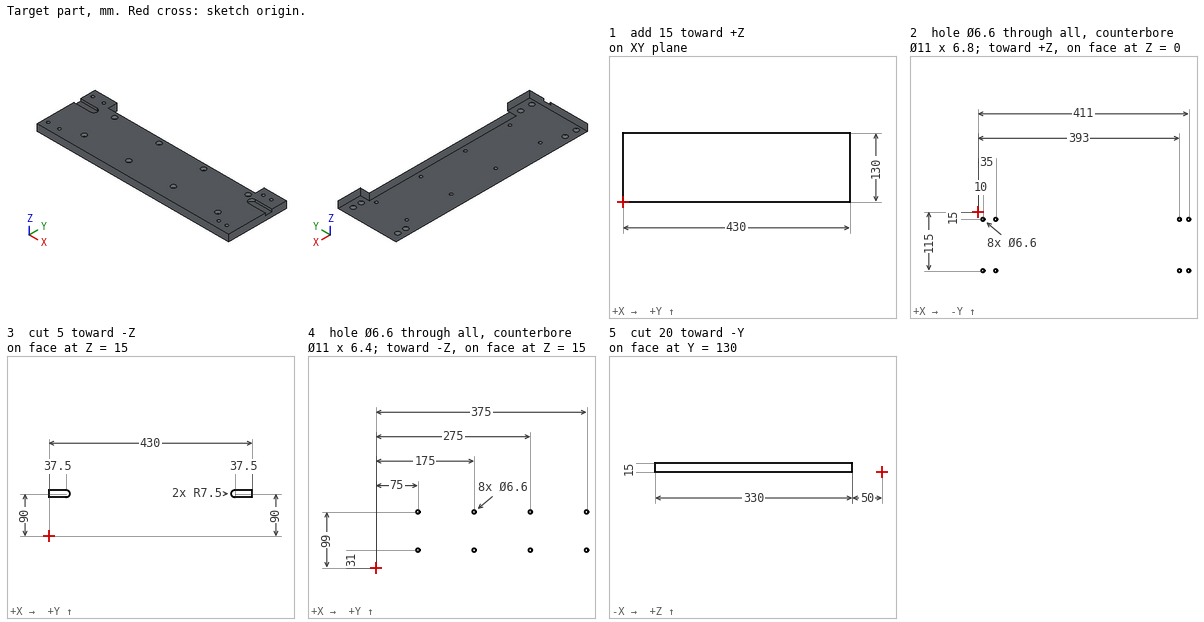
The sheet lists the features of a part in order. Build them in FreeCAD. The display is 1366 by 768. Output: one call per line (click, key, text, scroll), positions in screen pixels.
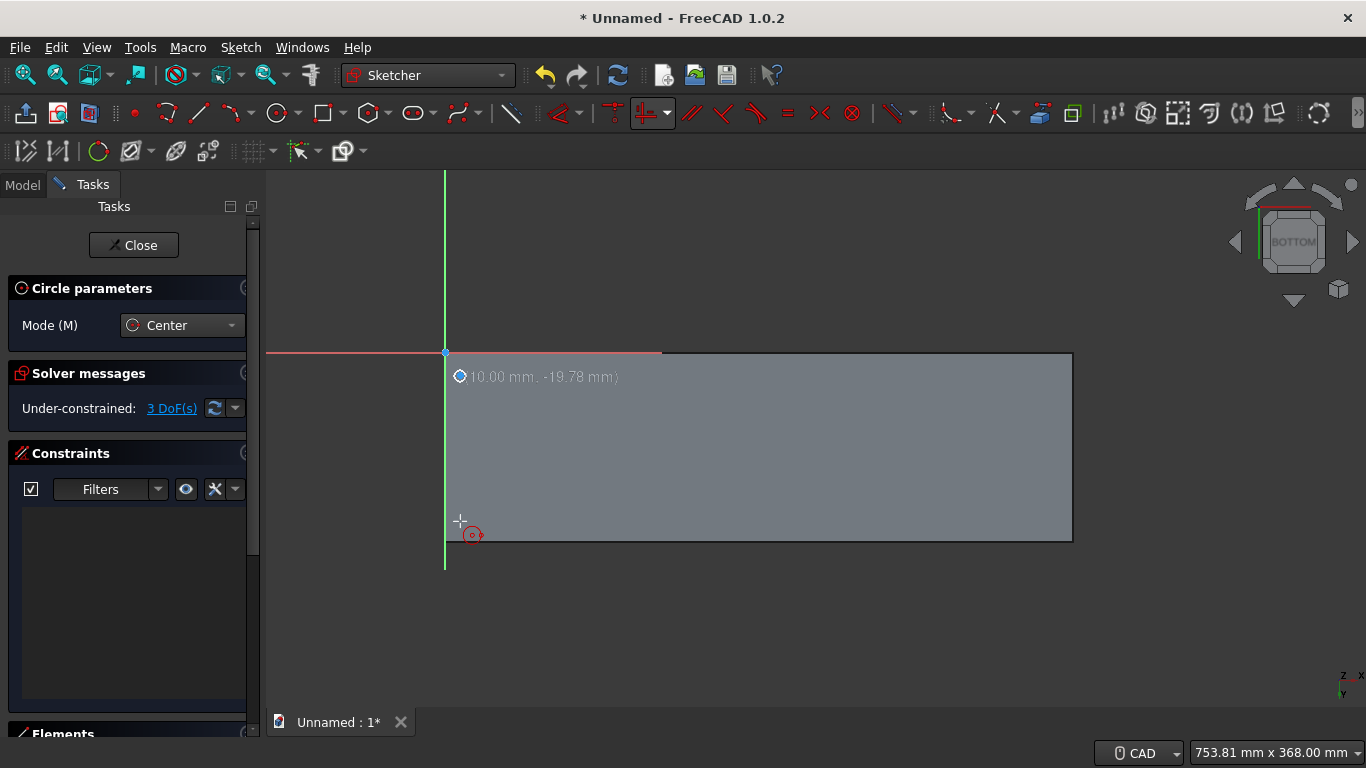
click(460, 521)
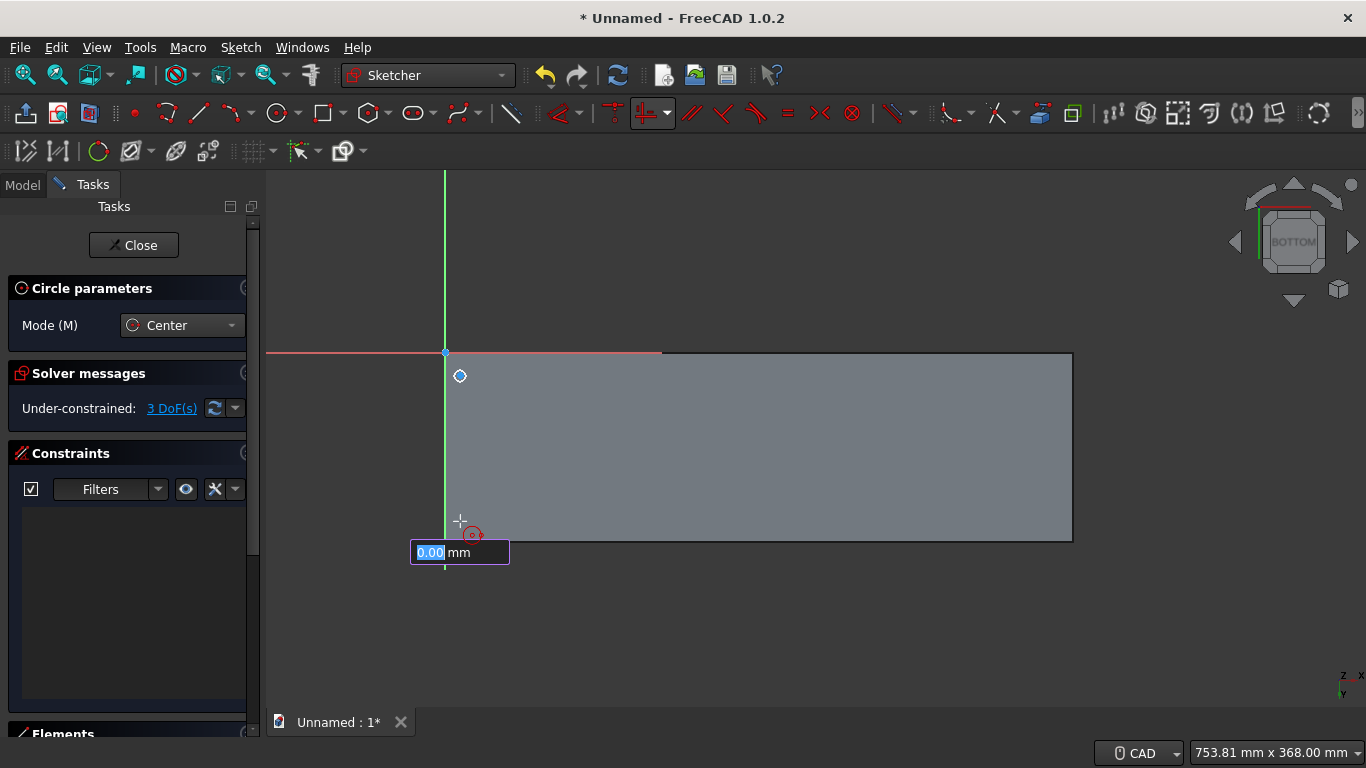
scroll(463, 517, up, 6)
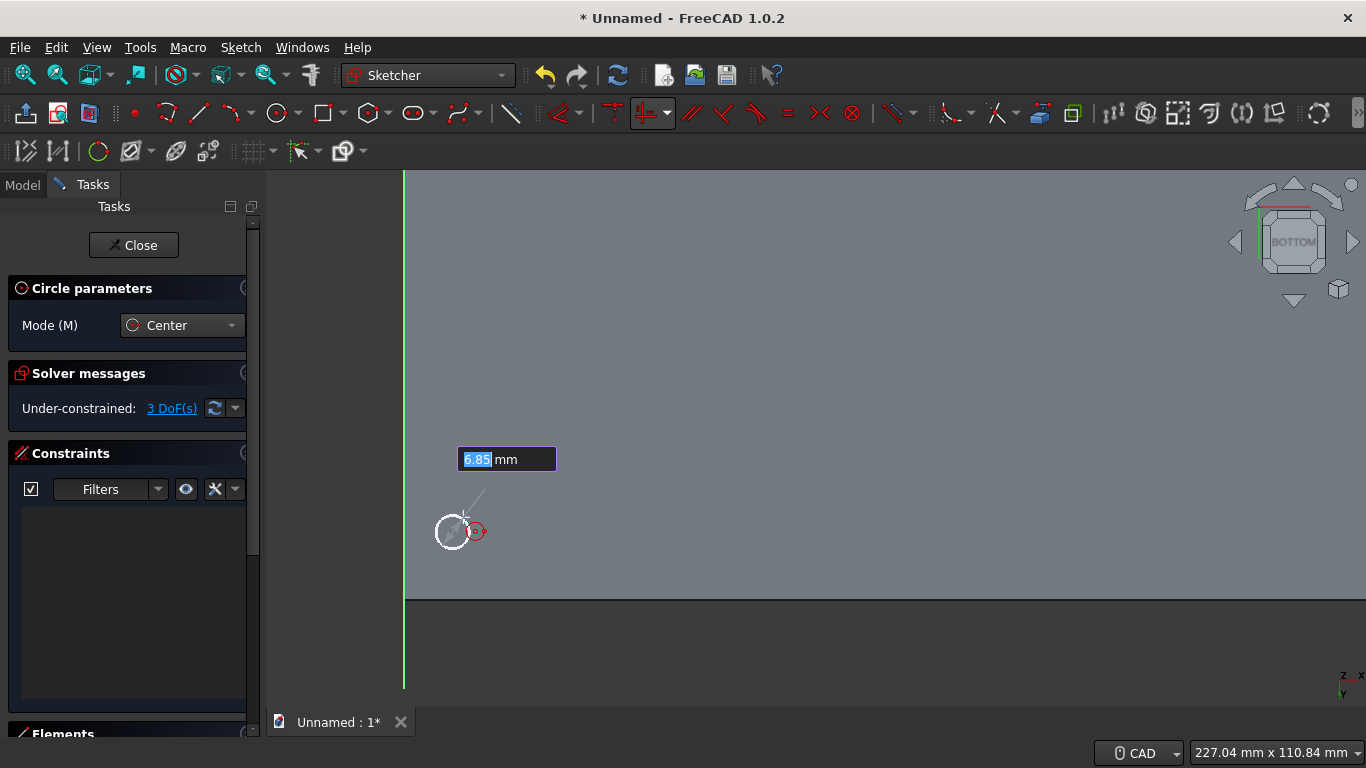
click(464, 516)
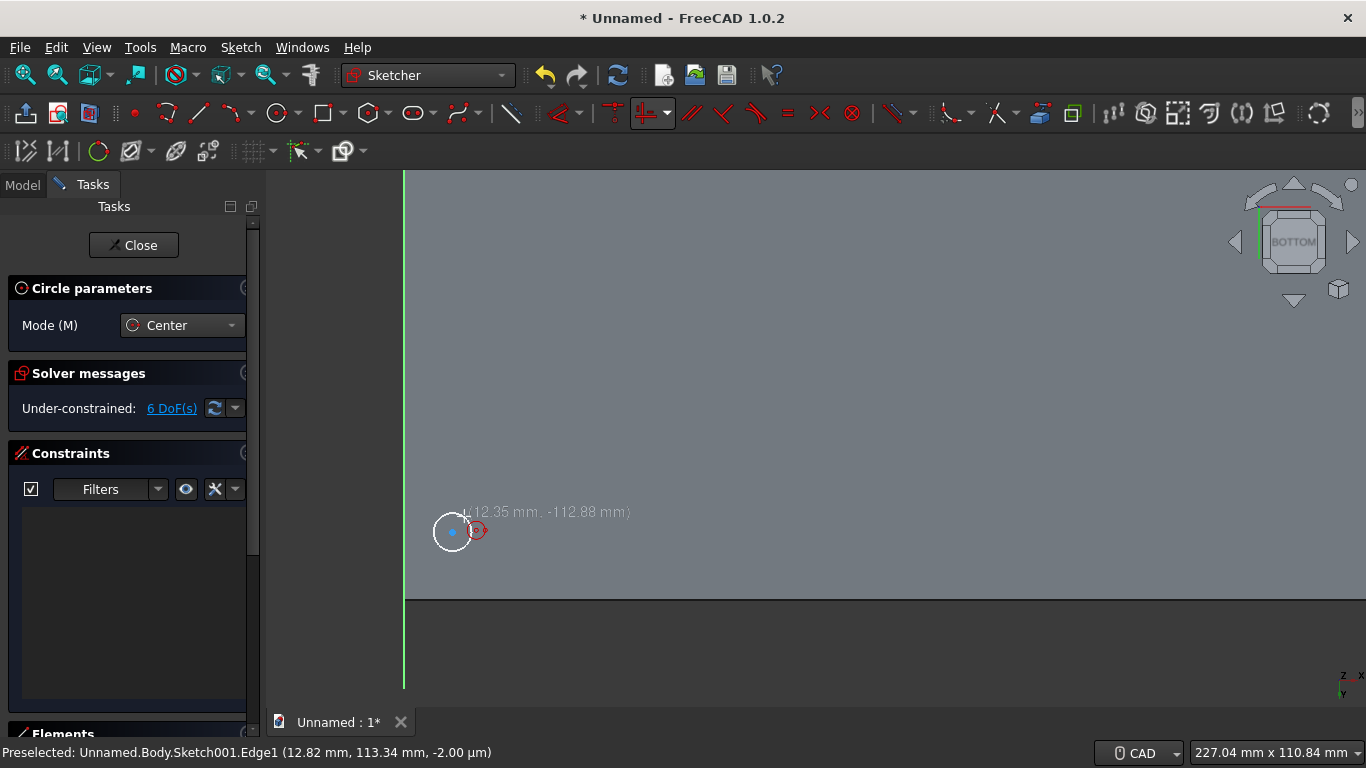
scroll(463, 517, down, 6)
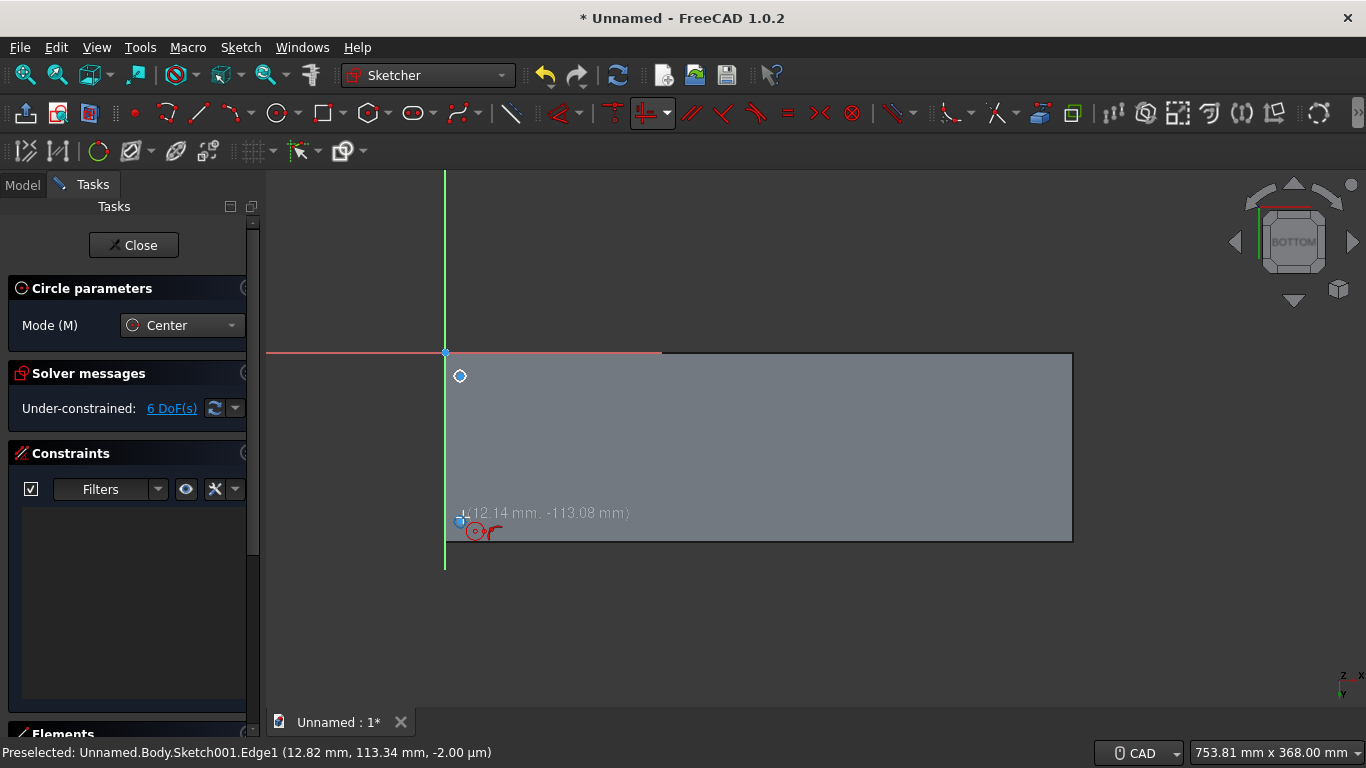
scroll(496, 375, up, 8)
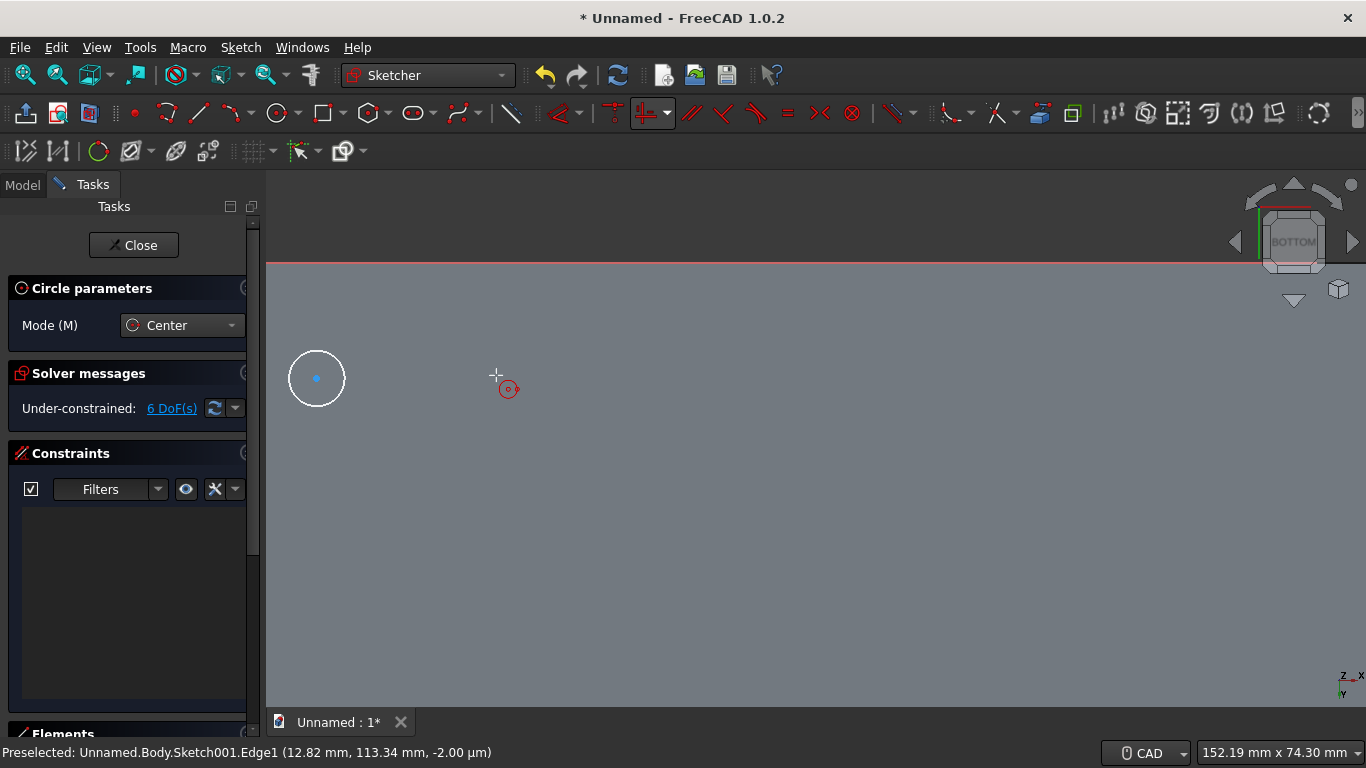
scroll(496, 375, down, 8)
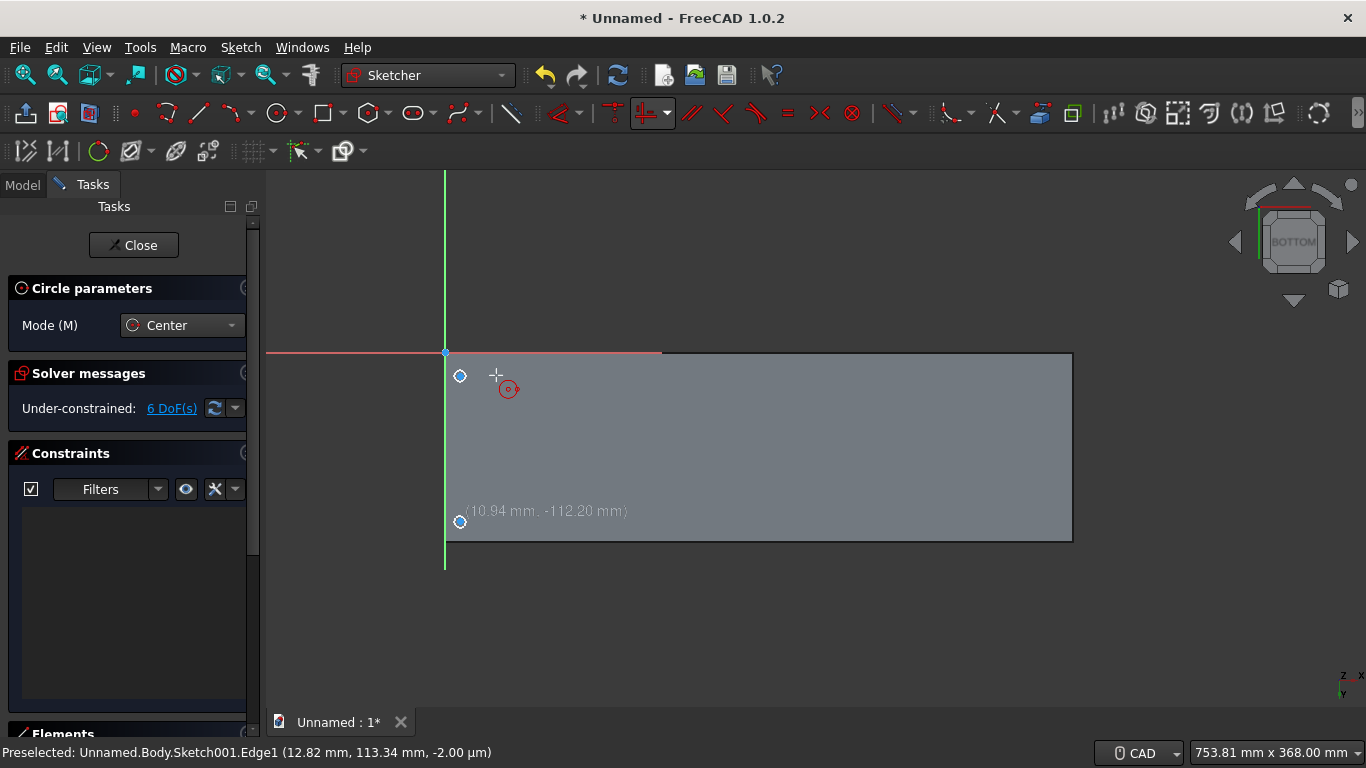
click(496, 375)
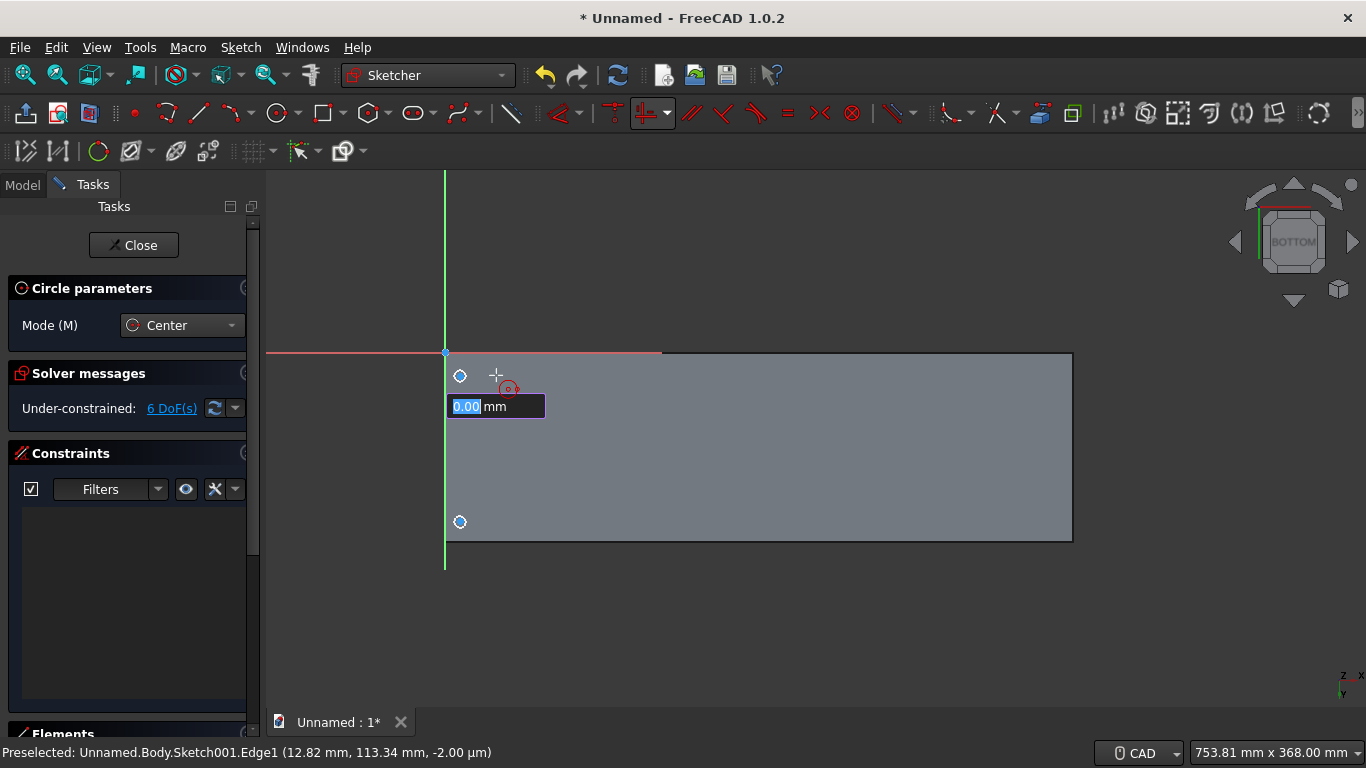
scroll(500, 371, up, 6)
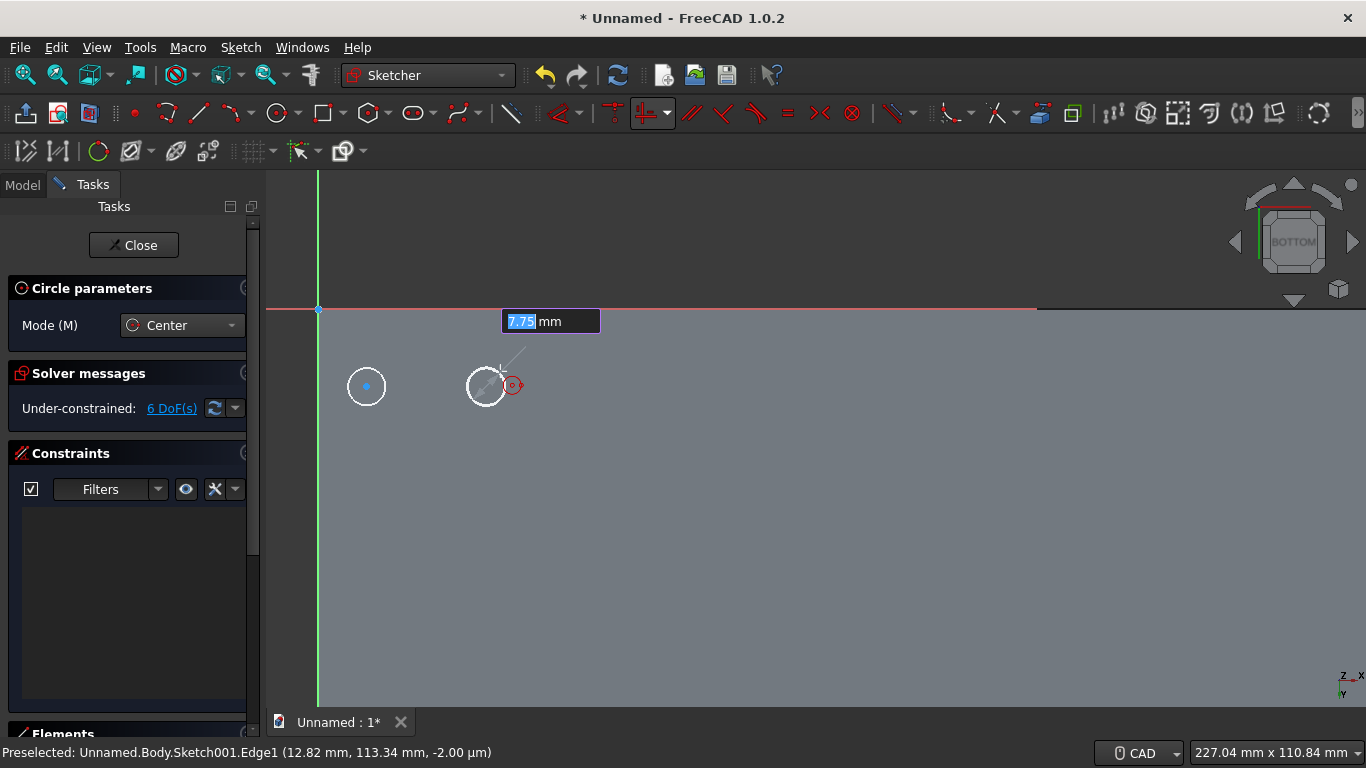
click(499, 371)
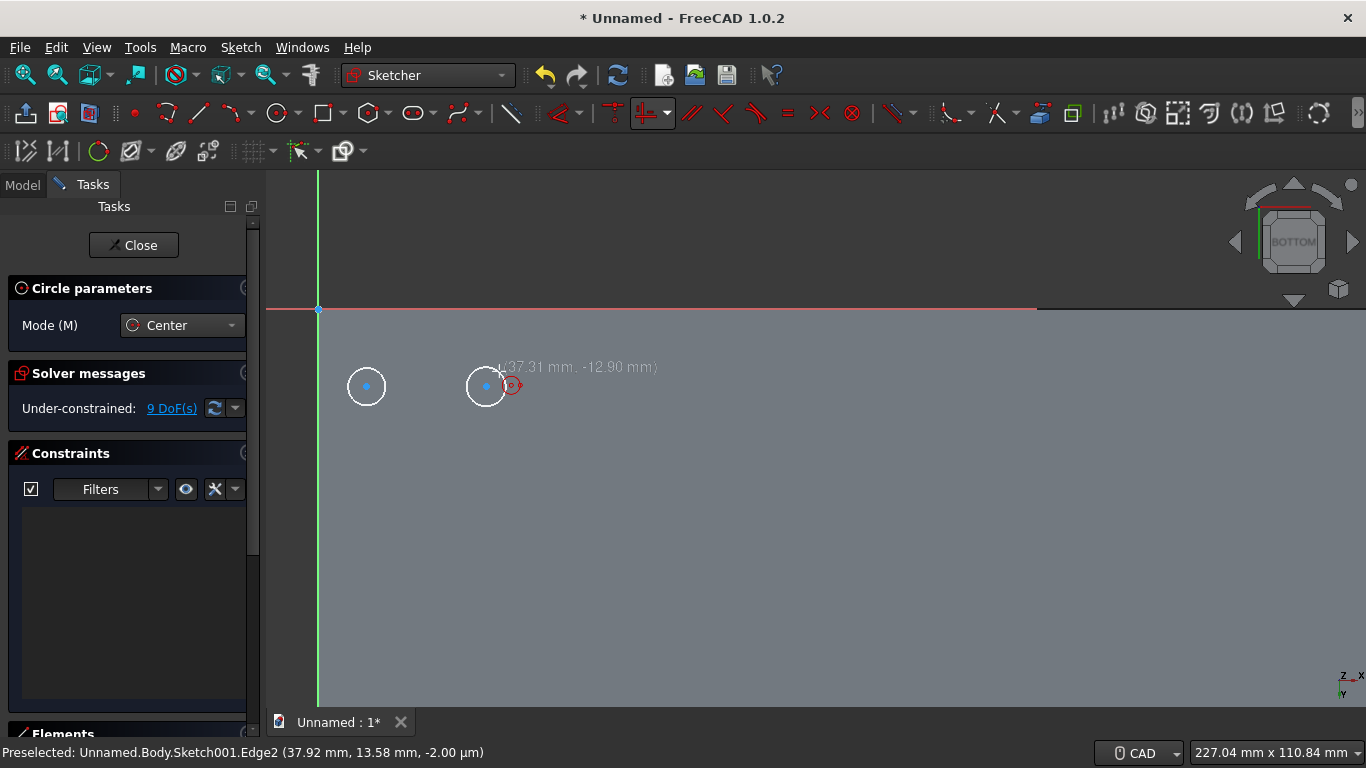
scroll(500, 371, down, 6)